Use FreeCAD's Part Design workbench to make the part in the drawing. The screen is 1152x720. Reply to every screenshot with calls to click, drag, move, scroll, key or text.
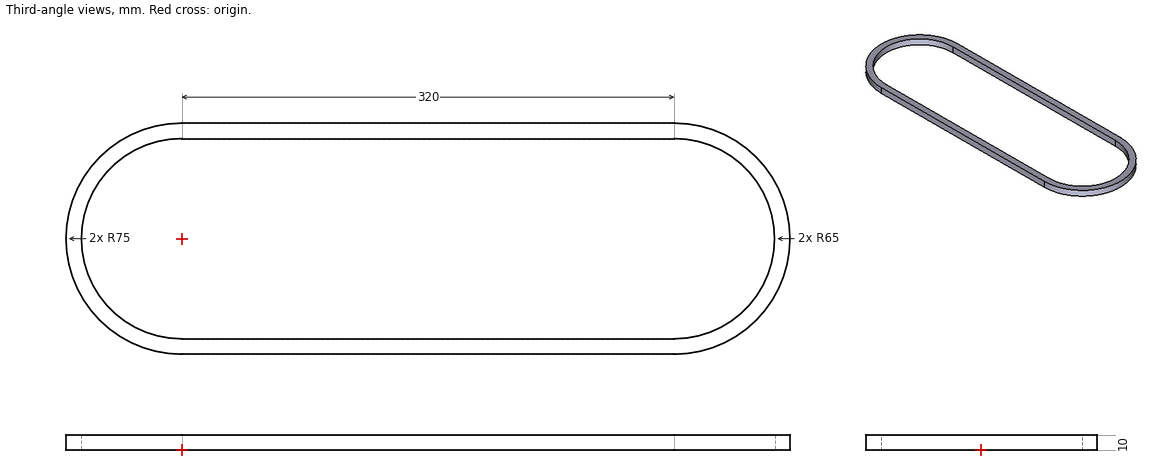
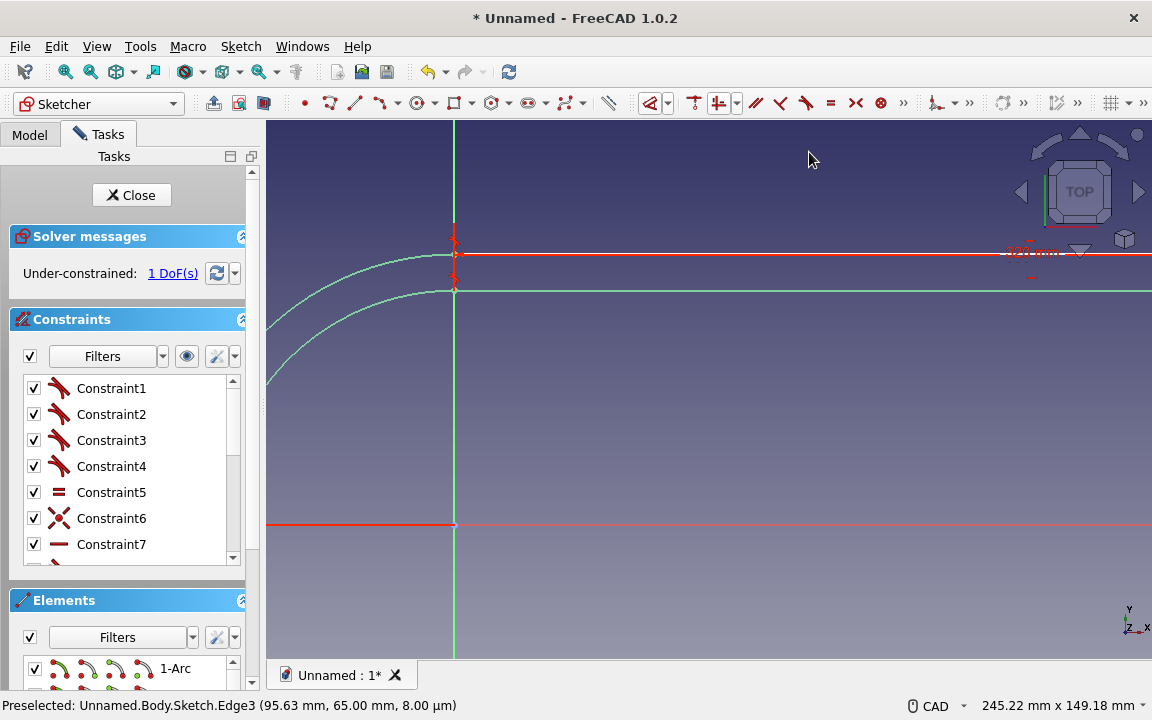
click(800, 254)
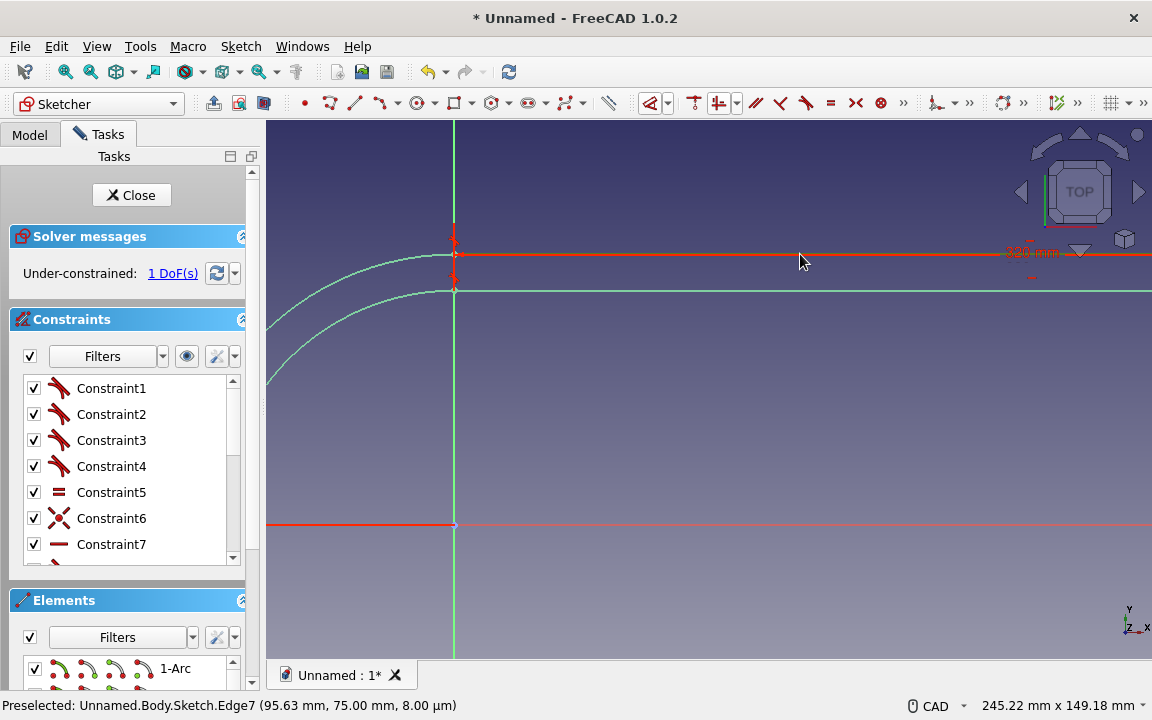
key(l)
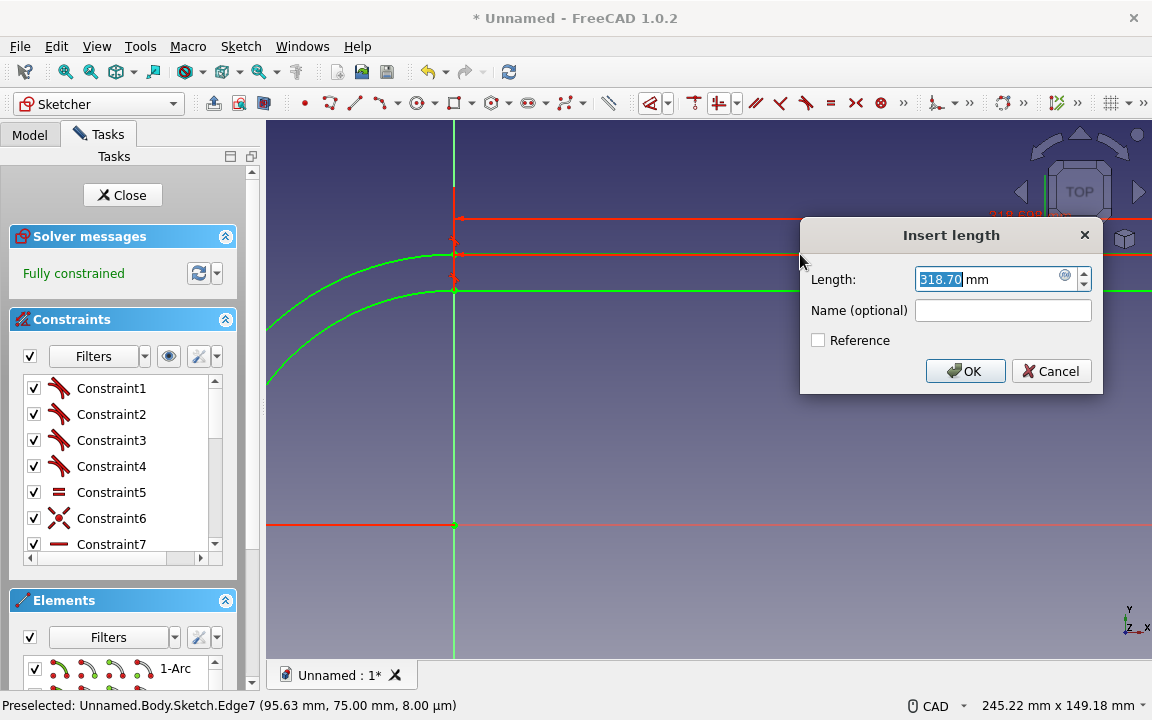
text(320)
key(Return)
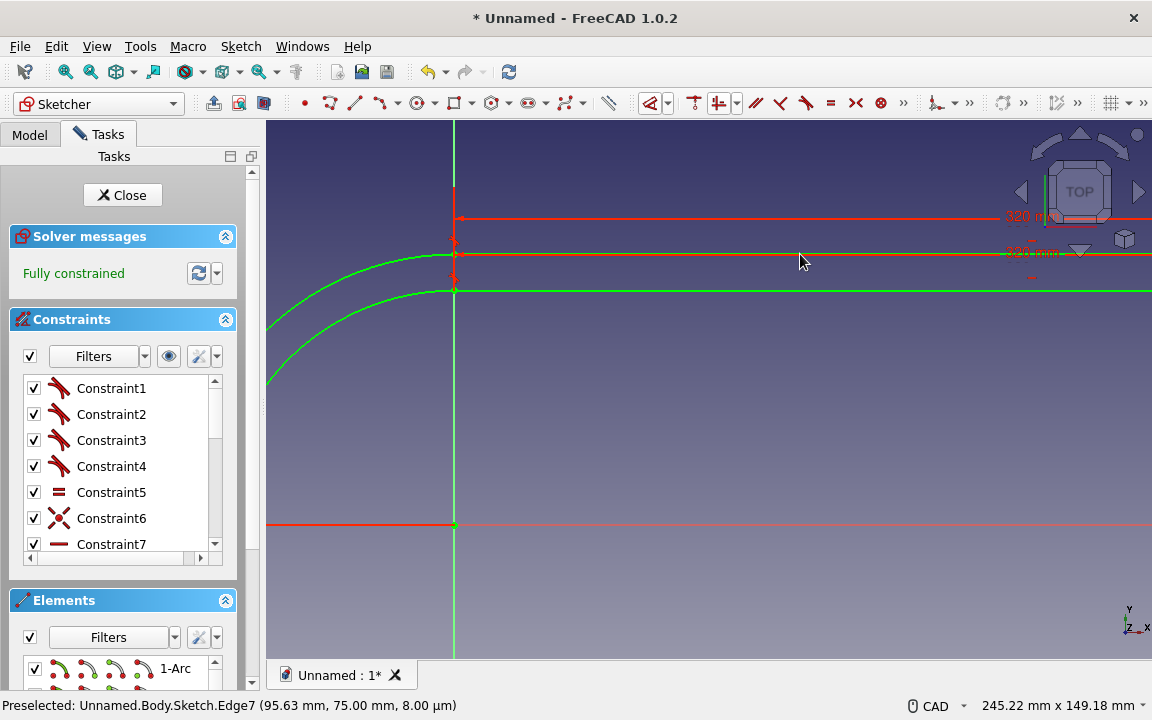
click(123, 195)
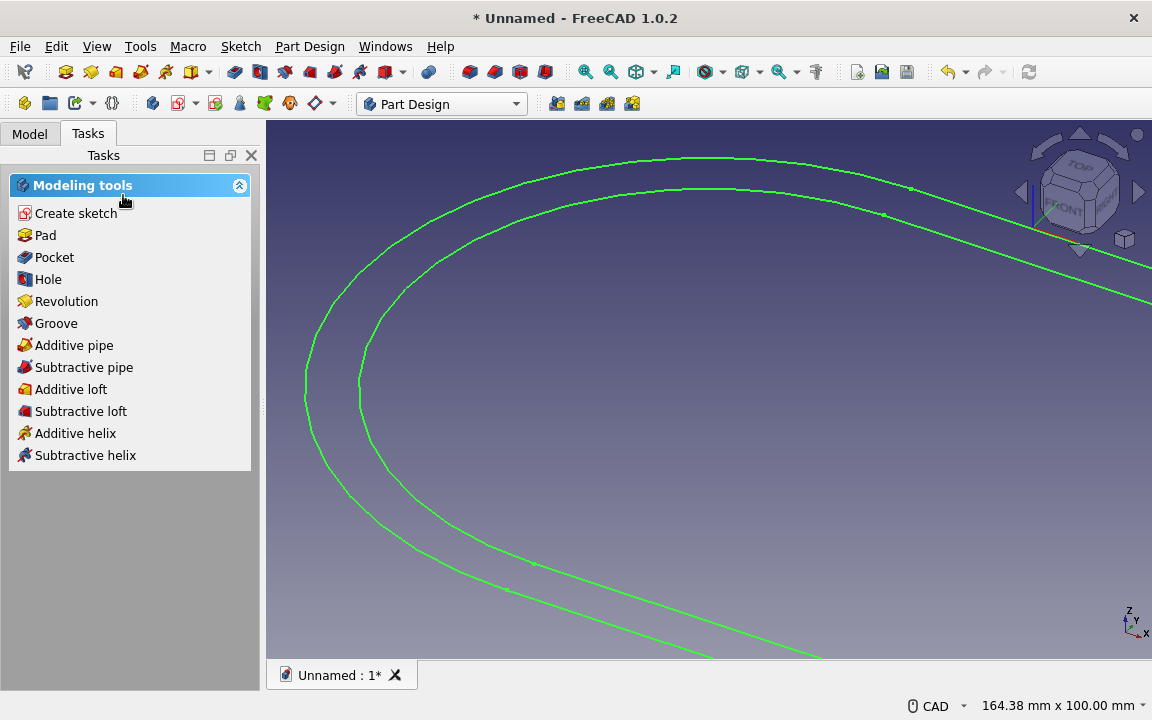
click(66, 72)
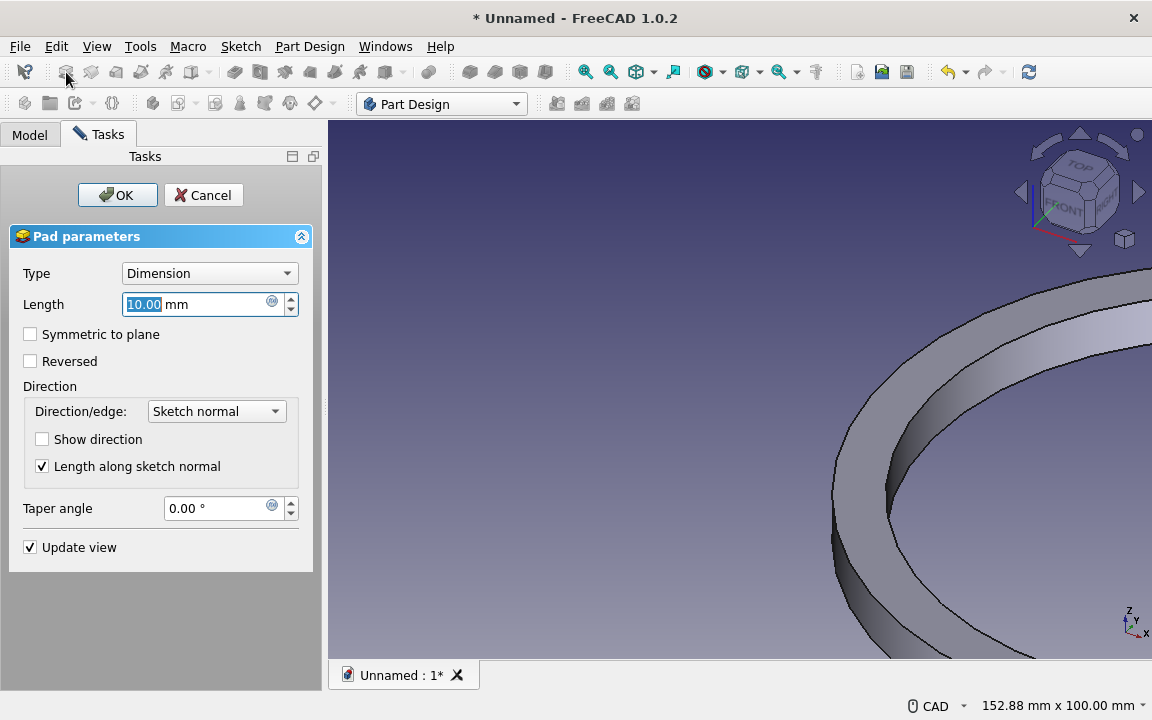
text(10)
key(Tab)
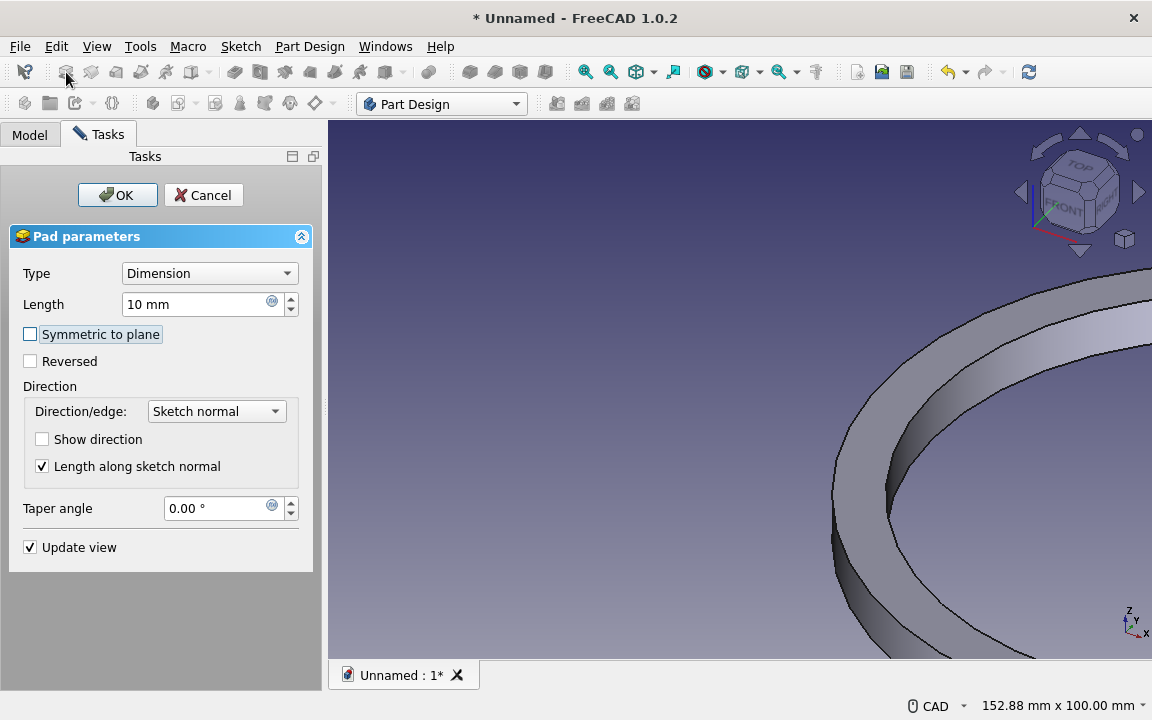
click(118, 195)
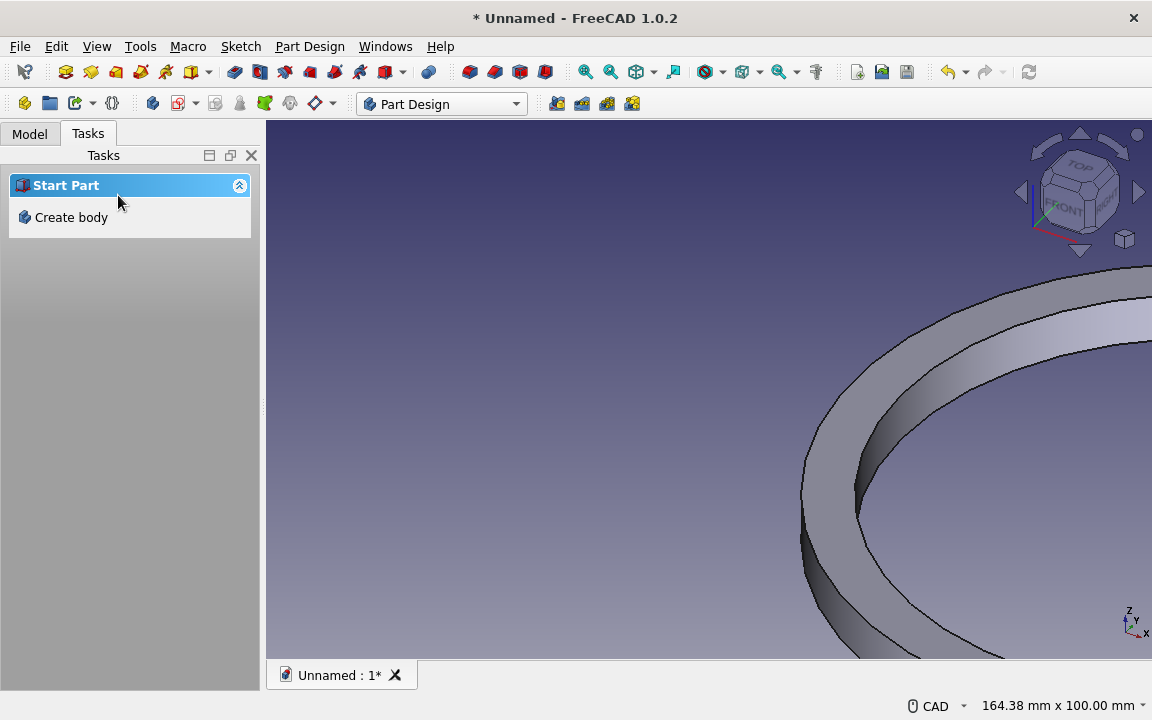
key(0)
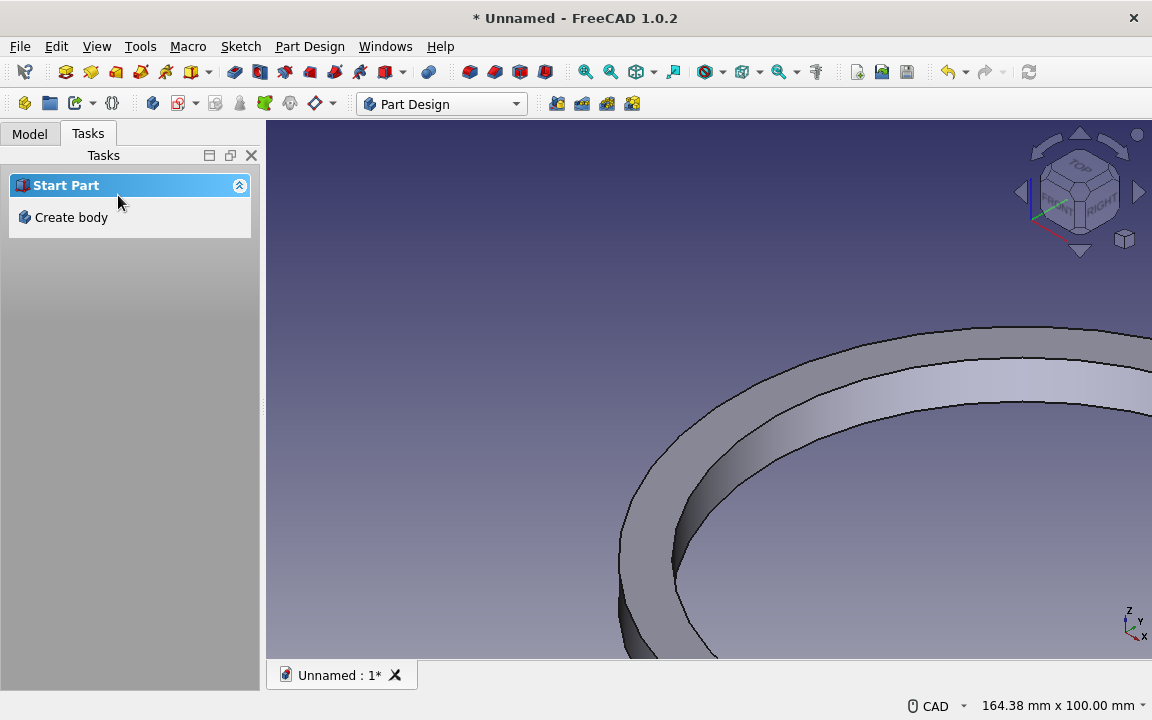
key(v)
key(f)